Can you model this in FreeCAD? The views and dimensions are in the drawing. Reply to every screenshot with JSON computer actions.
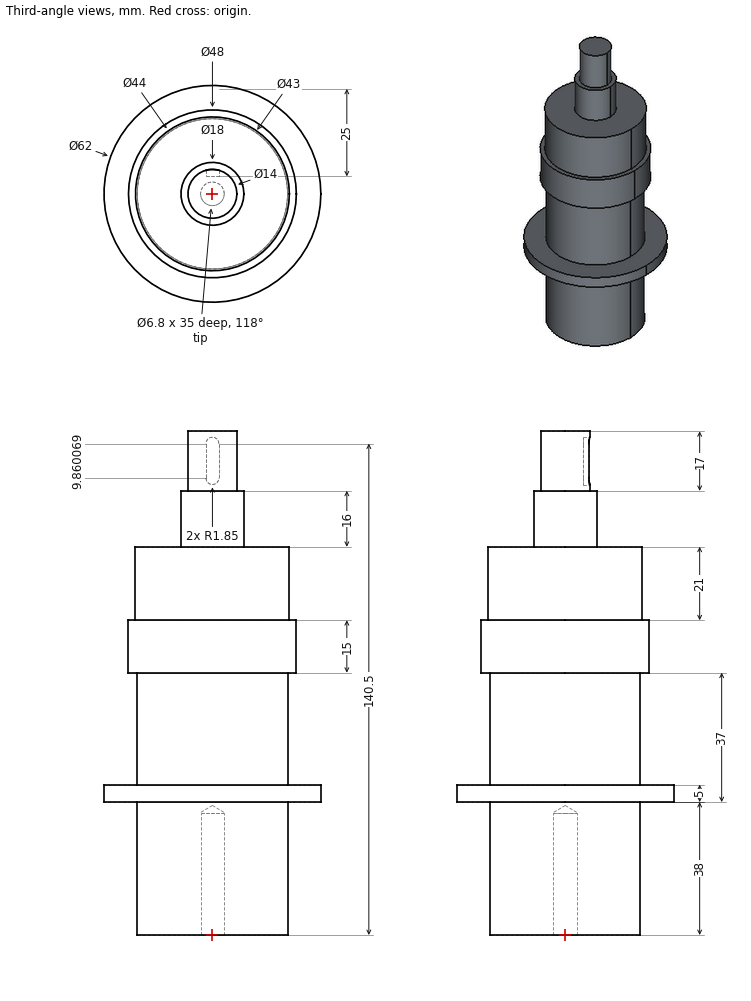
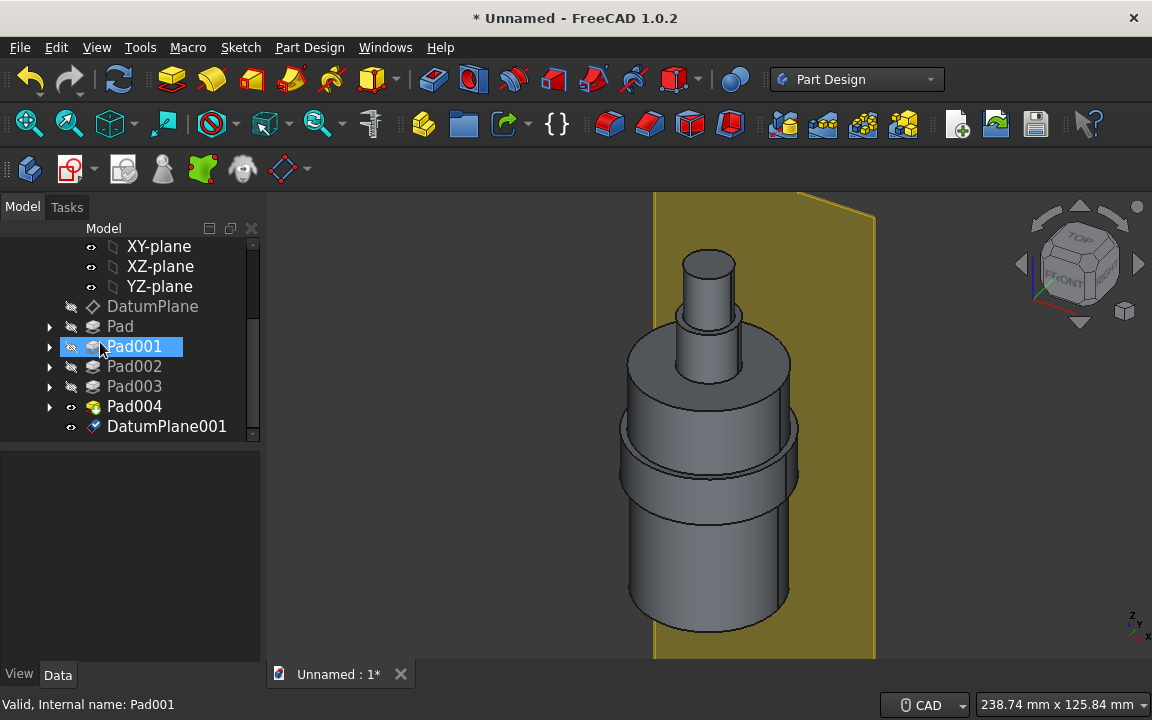
{"action": "left_click", "coordinate": [116, 427]}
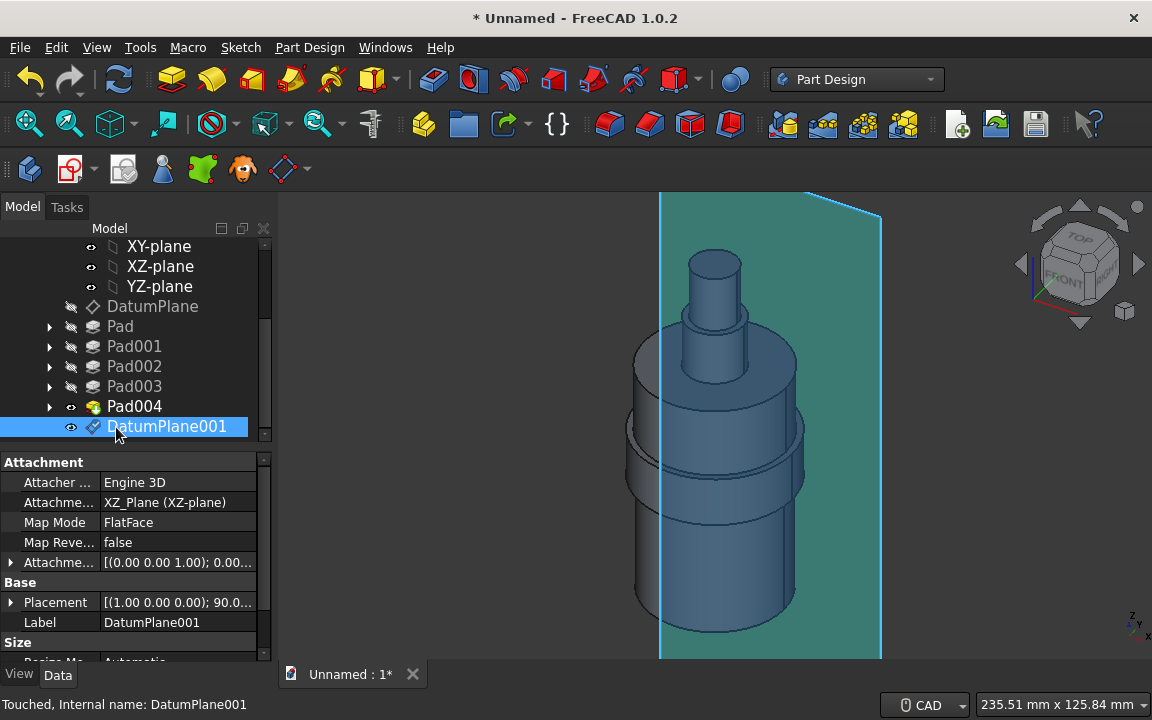
{"action": "left_click", "coordinate": [70, 170]}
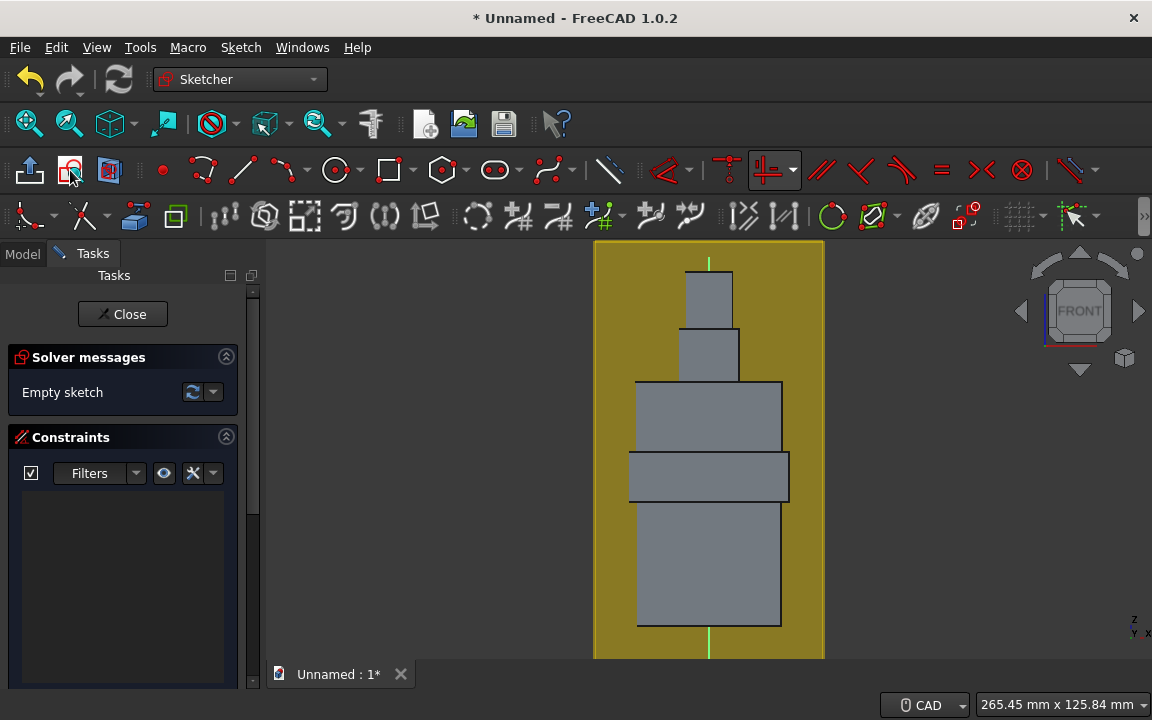
{"action": "left_click", "coordinate": [110, 170]}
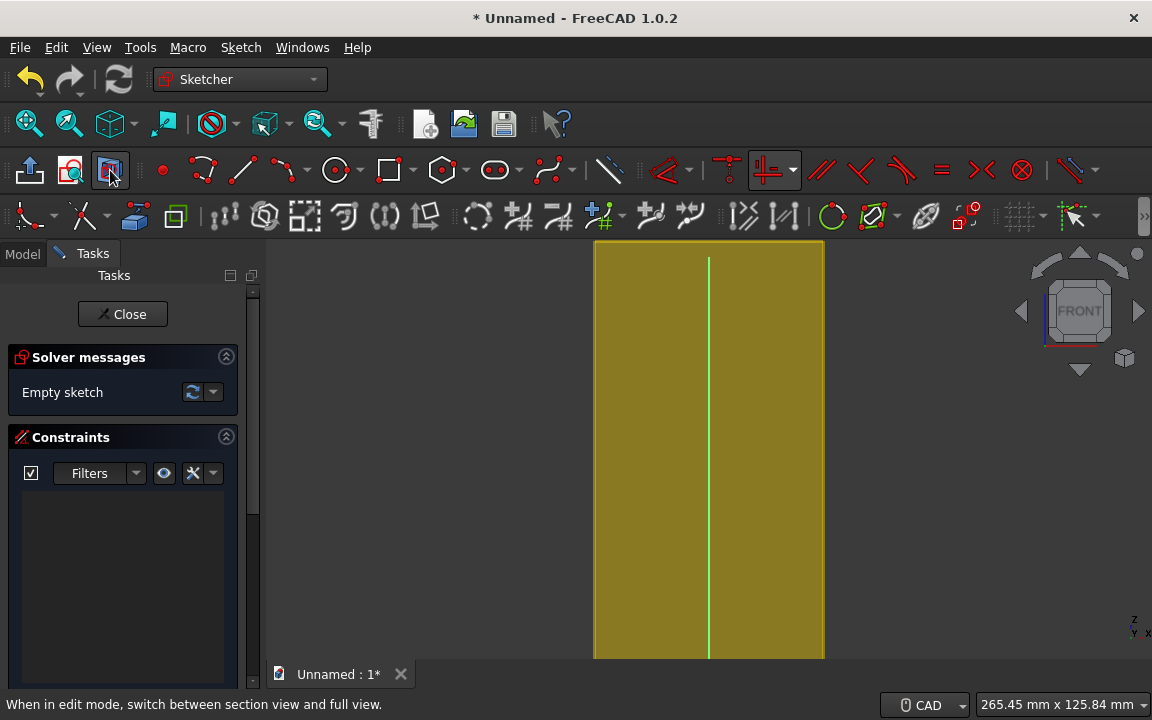
{"action": "scroll", "coordinate": [722, 271], "scroll_direction": "up", "scroll_amount": 9}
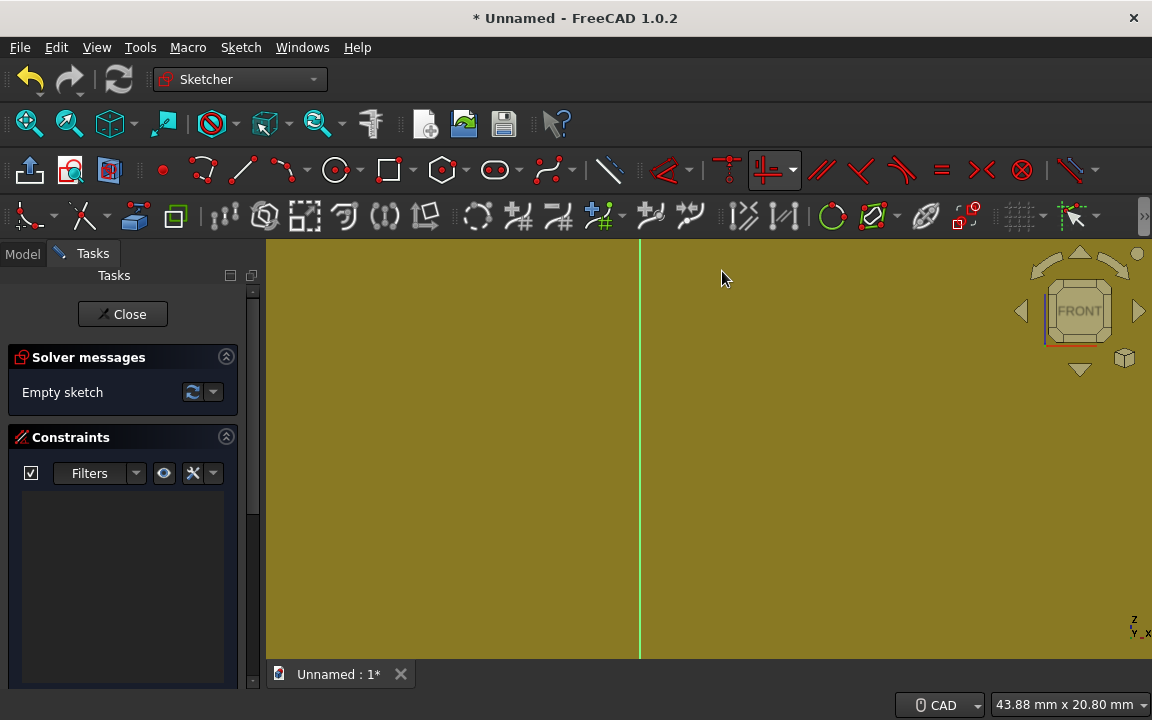
{"action": "left_click", "coordinate": [496, 170]}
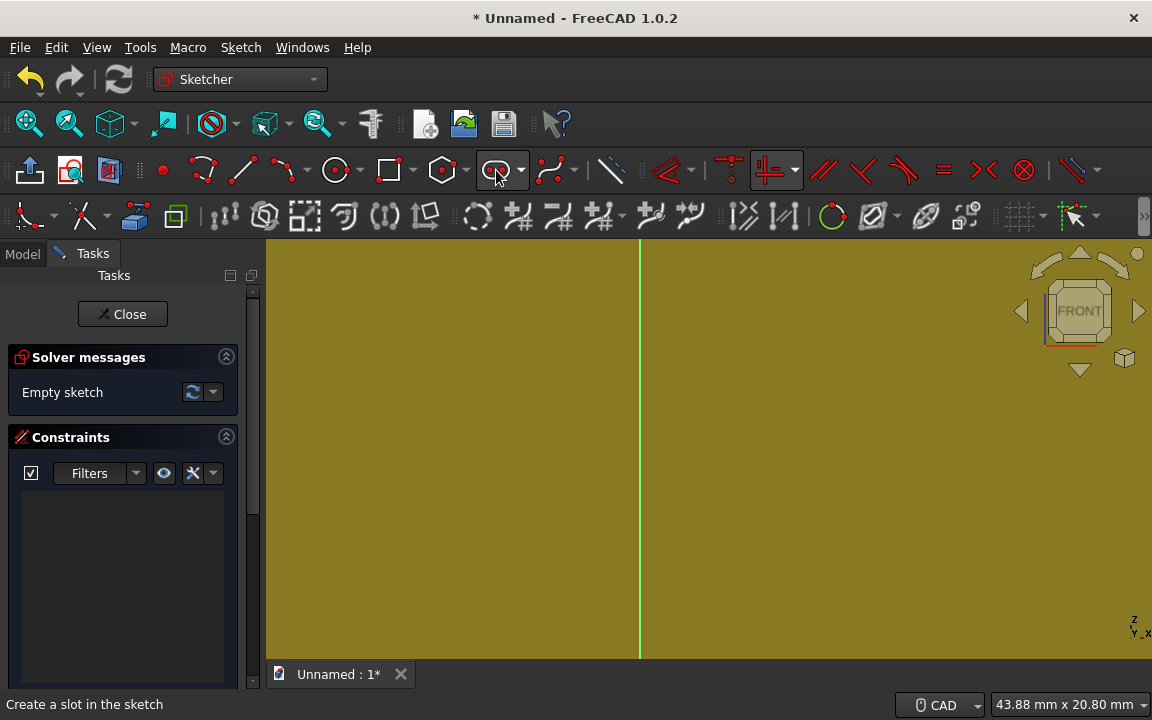
{"action": "left_click", "coordinate": [640, 547]}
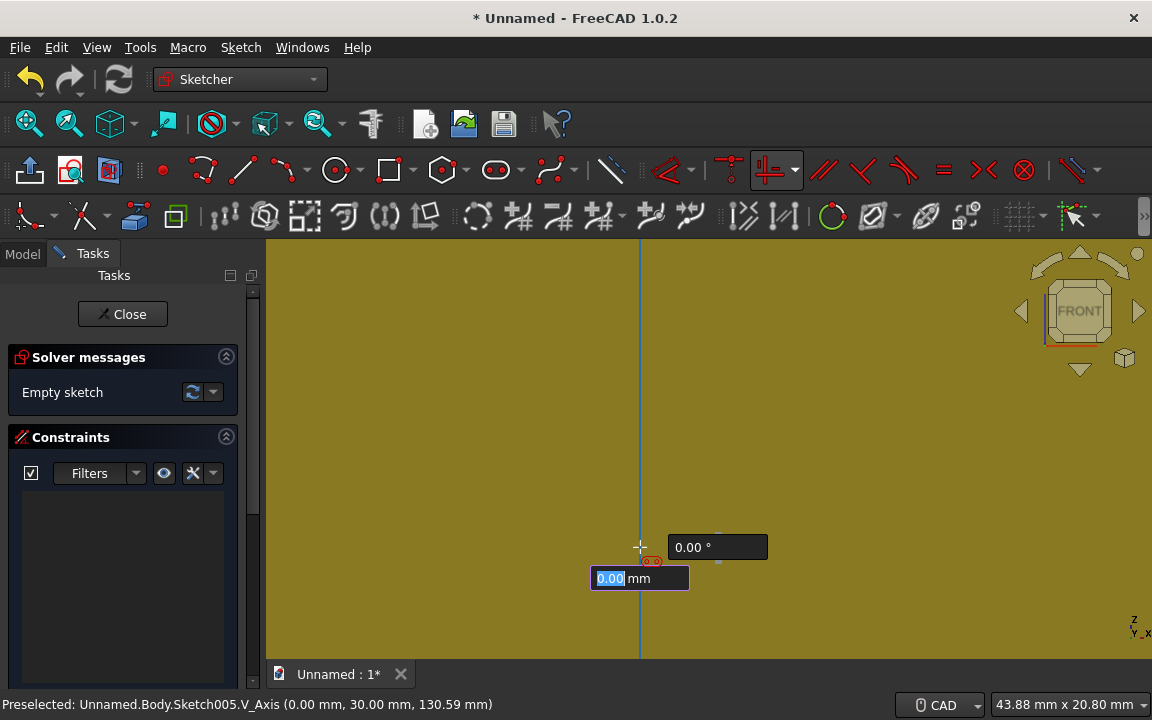
{"action": "left_click", "coordinate": [649, 348]}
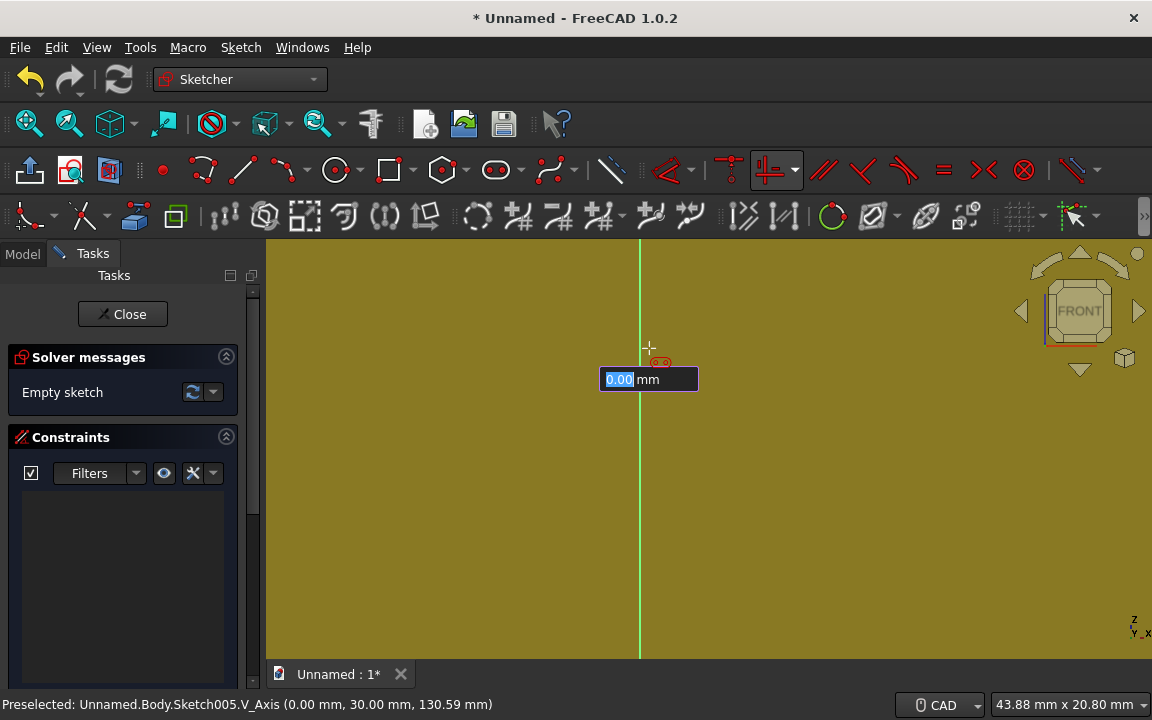
{"action": "left_click", "coordinate": [677, 448]}
{"action": "key", "text": "Escape"}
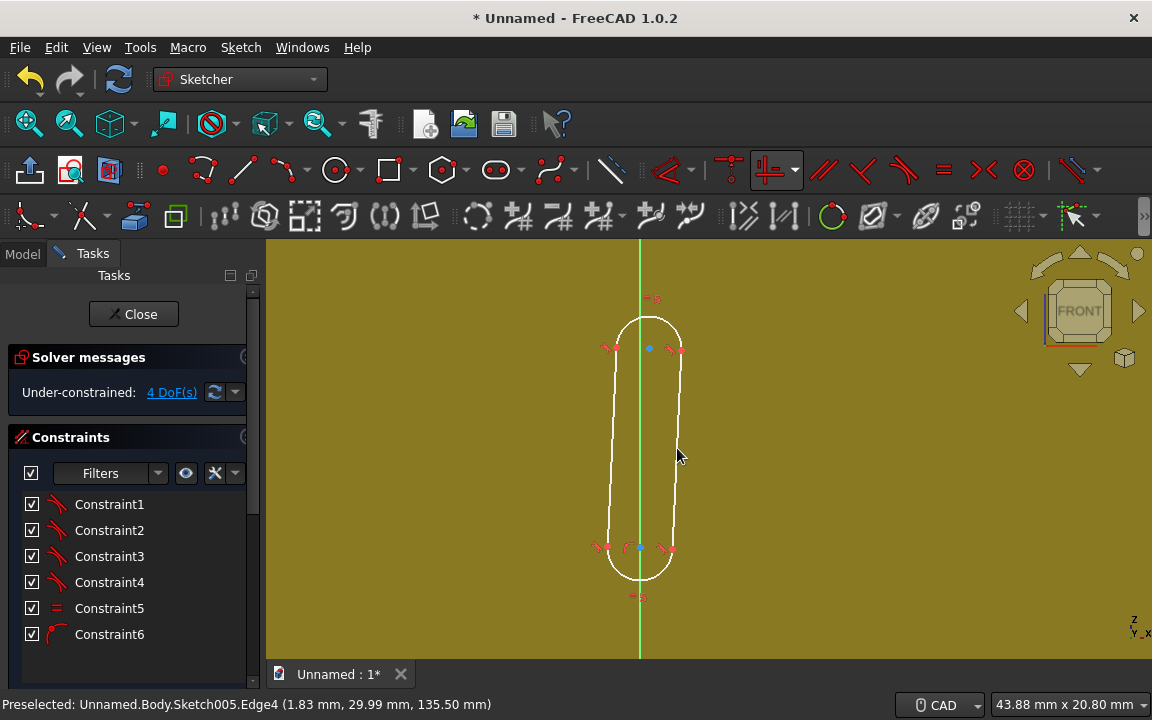
{"action": "left_click", "coordinate": [610, 487]}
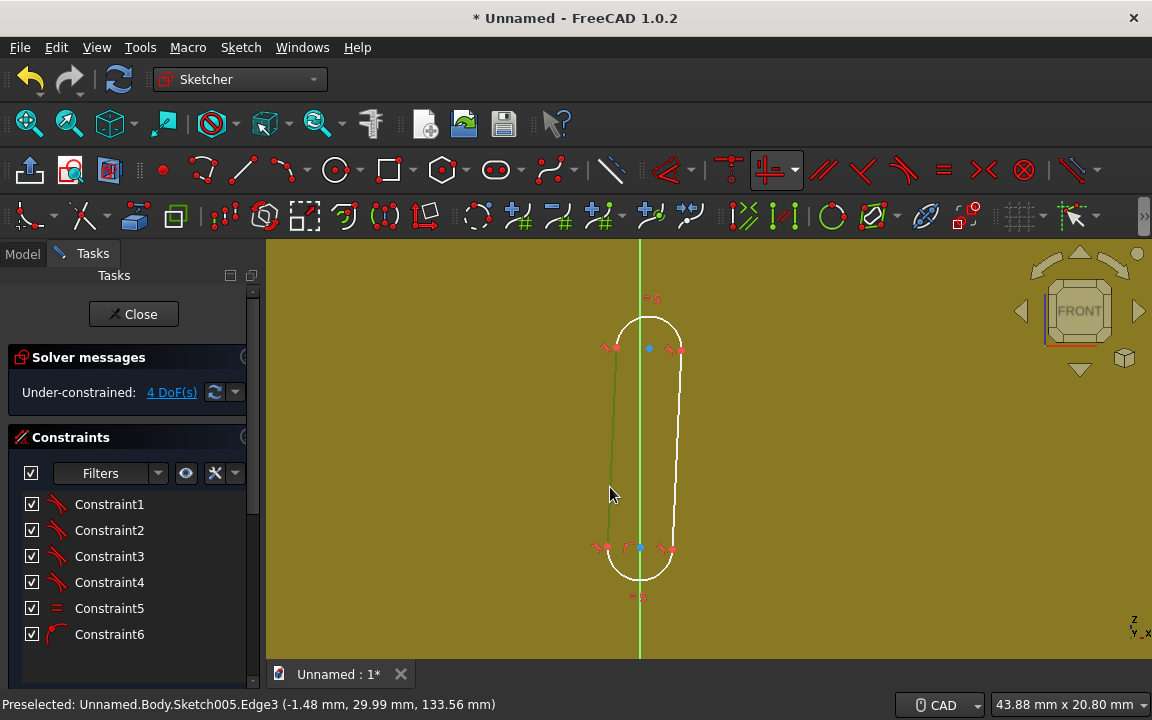
{"action": "left_click", "coordinate": [798, 170]}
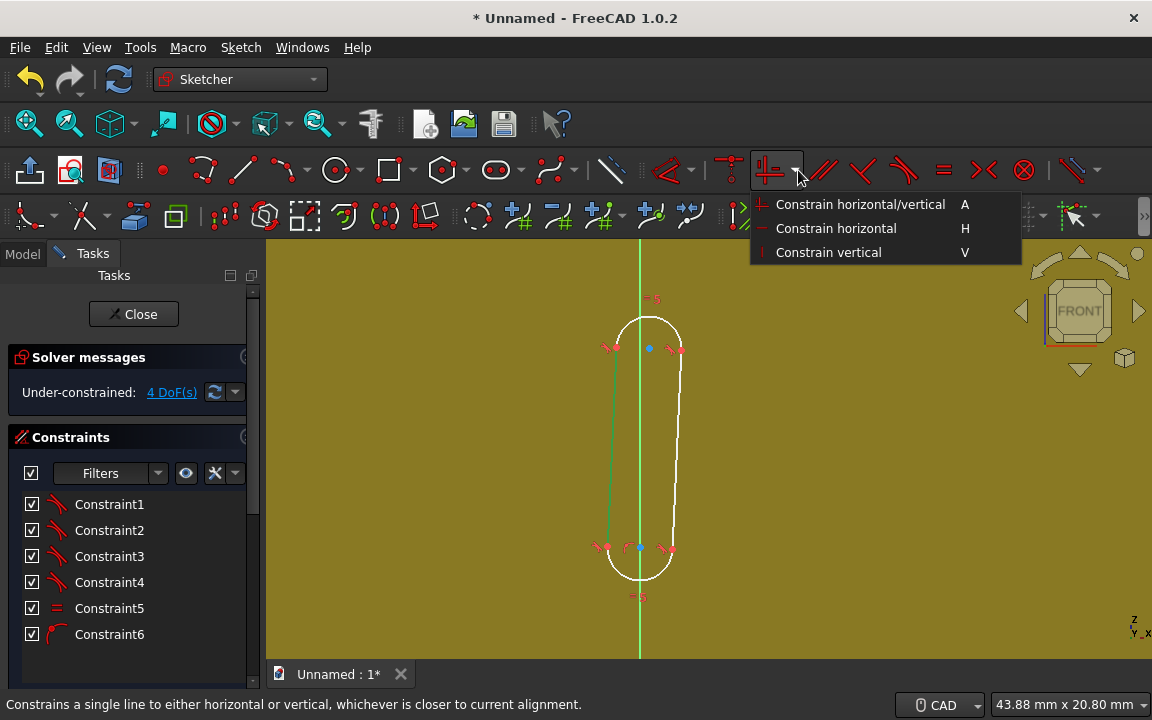
{"action": "left_click", "coordinate": [886, 252]}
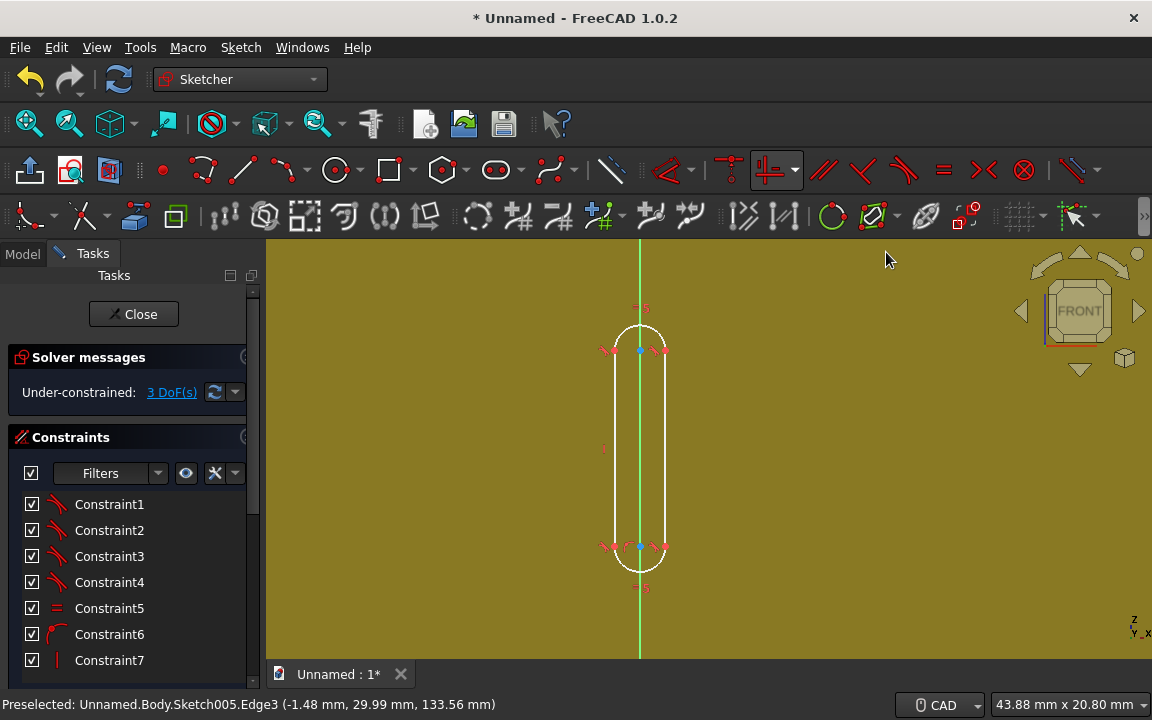
{"action": "left_click", "coordinate": [666, 170]}